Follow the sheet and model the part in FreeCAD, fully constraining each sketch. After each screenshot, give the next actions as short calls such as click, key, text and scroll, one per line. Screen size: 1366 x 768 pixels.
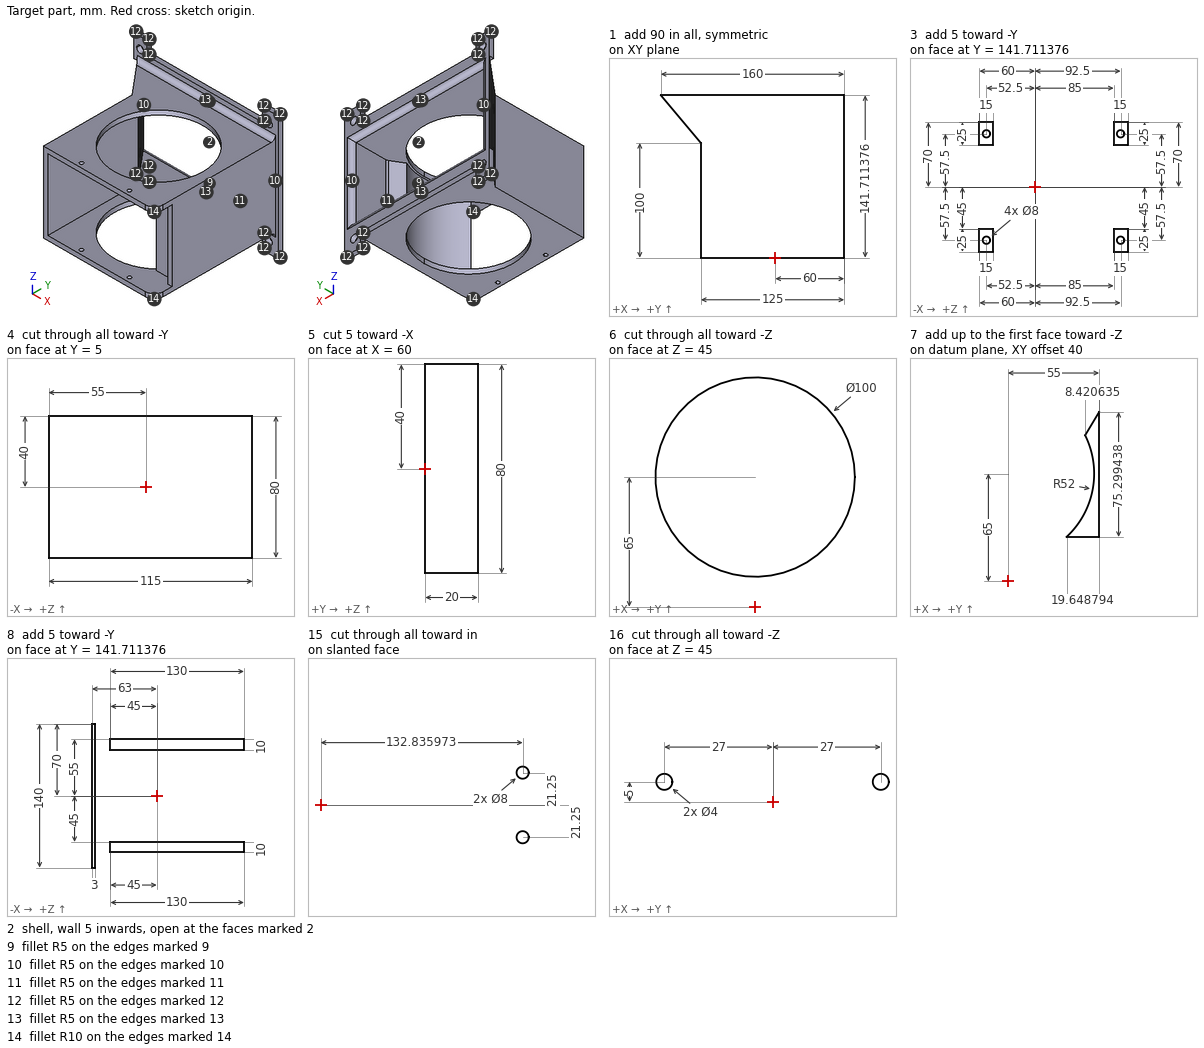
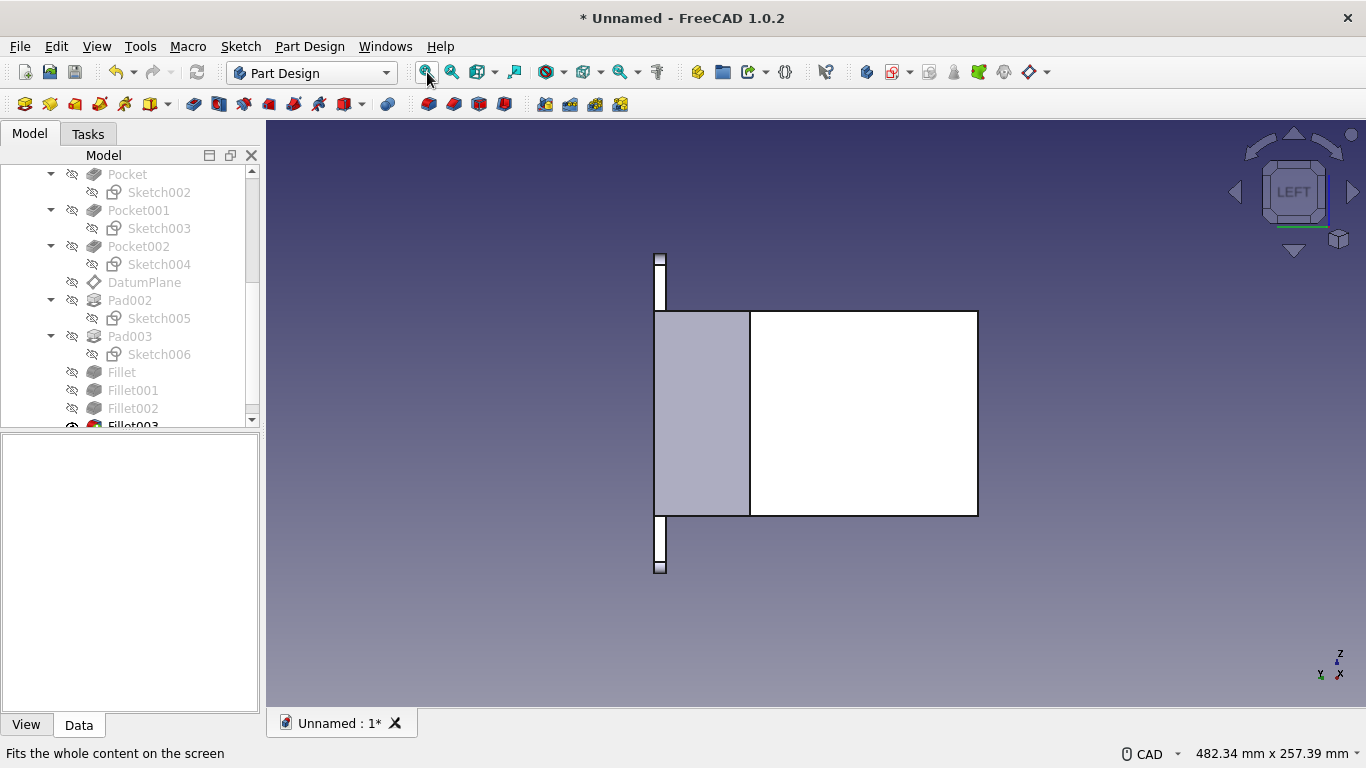
key(v)
key(3)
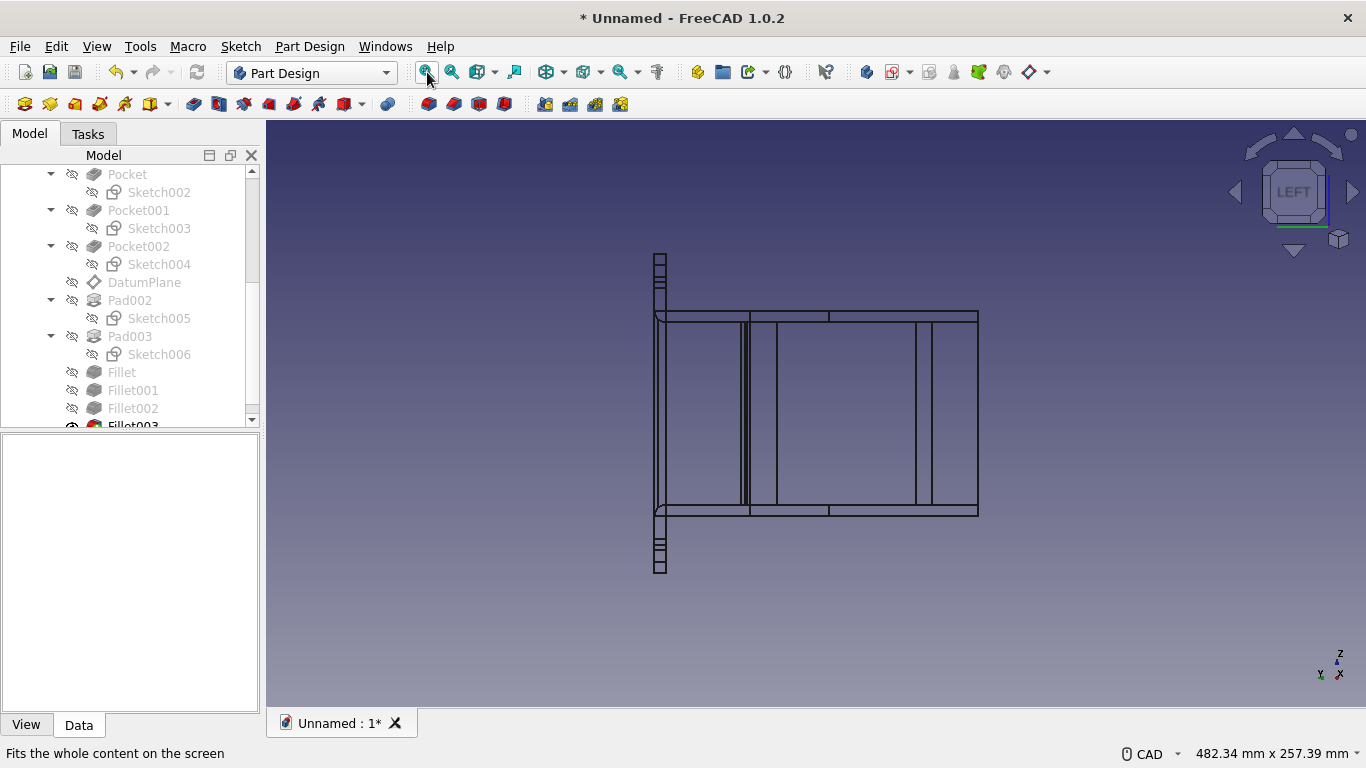
key(0)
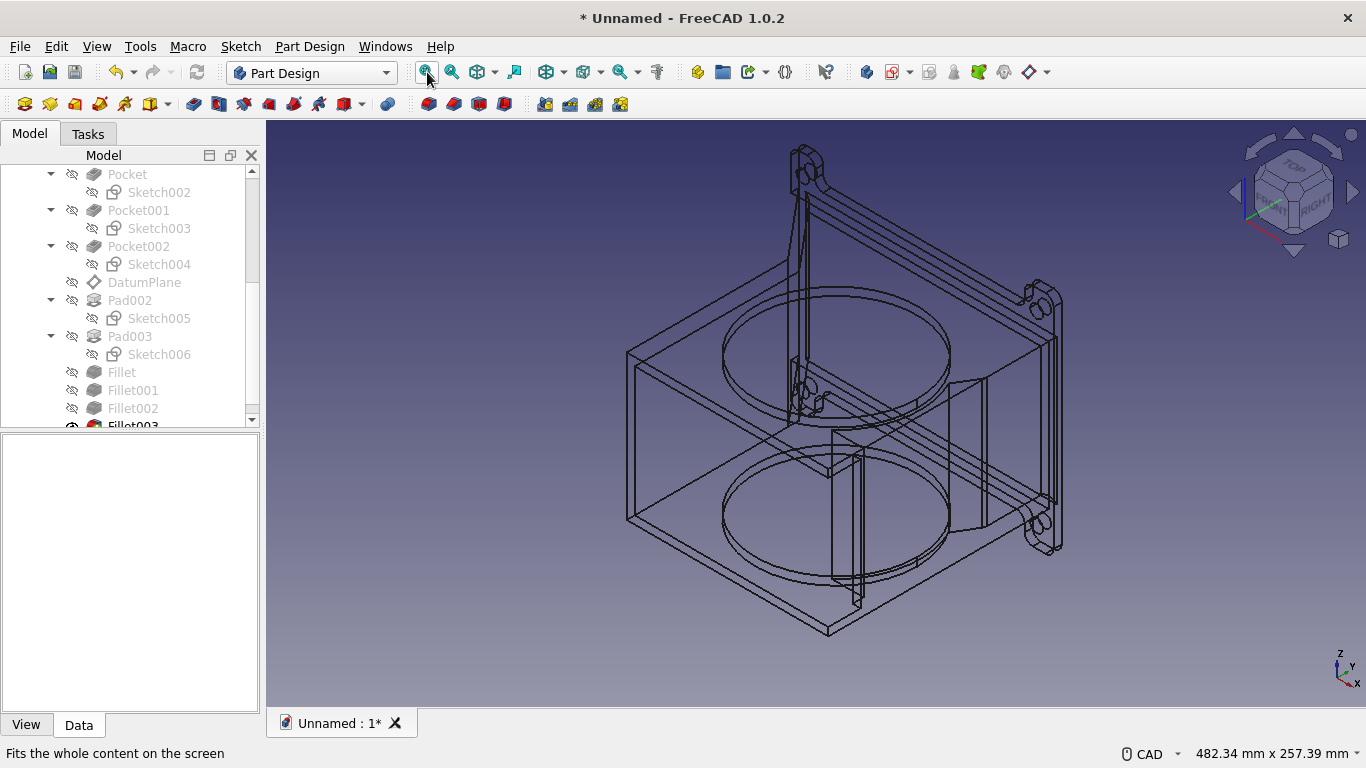
click(923, 436)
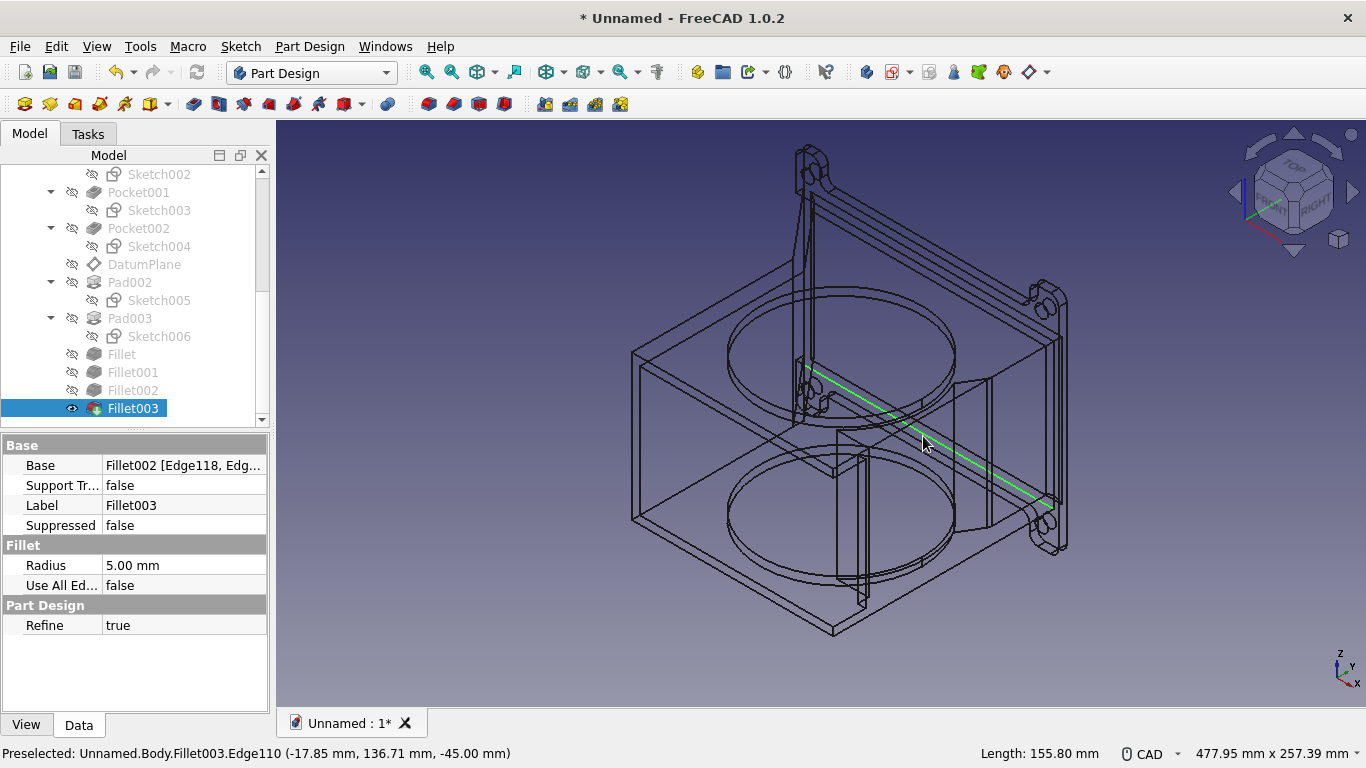
click(928, 268, ctrl)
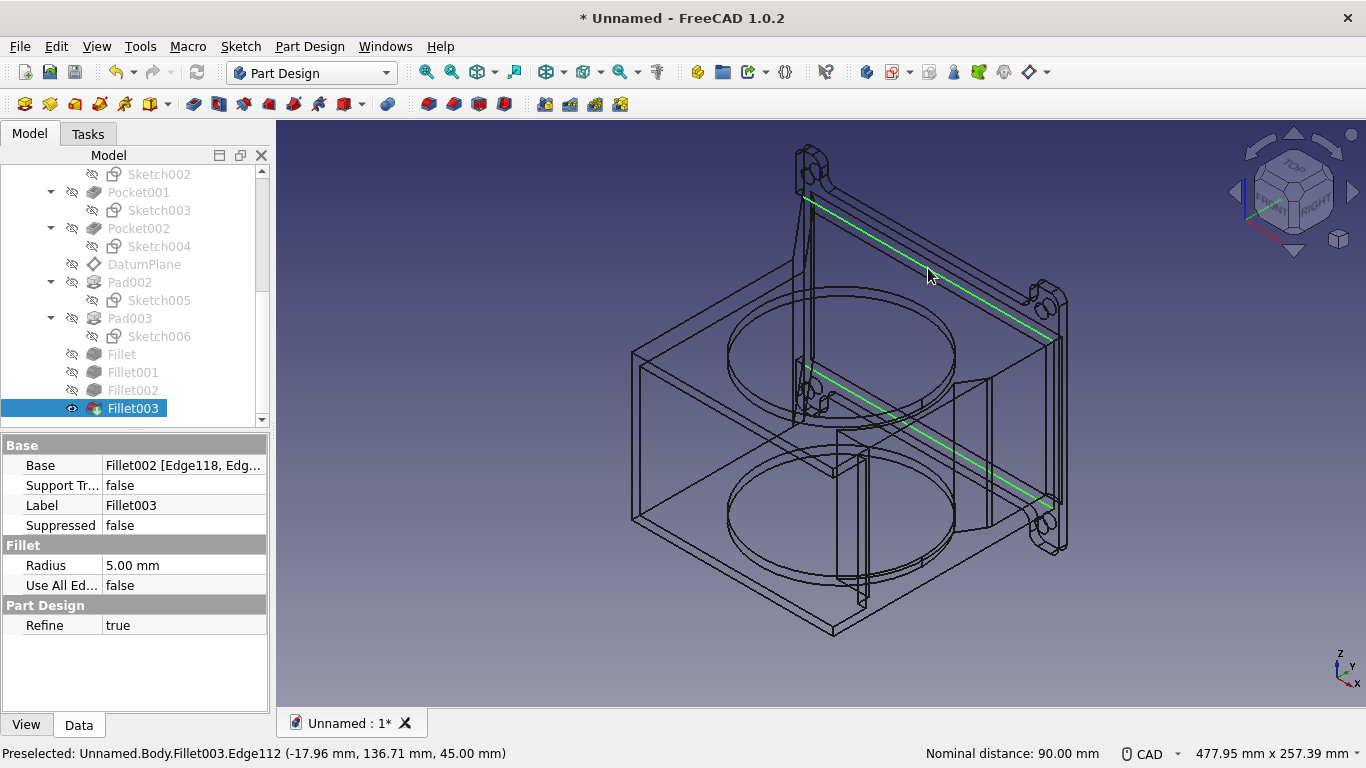
key(v)
key(1)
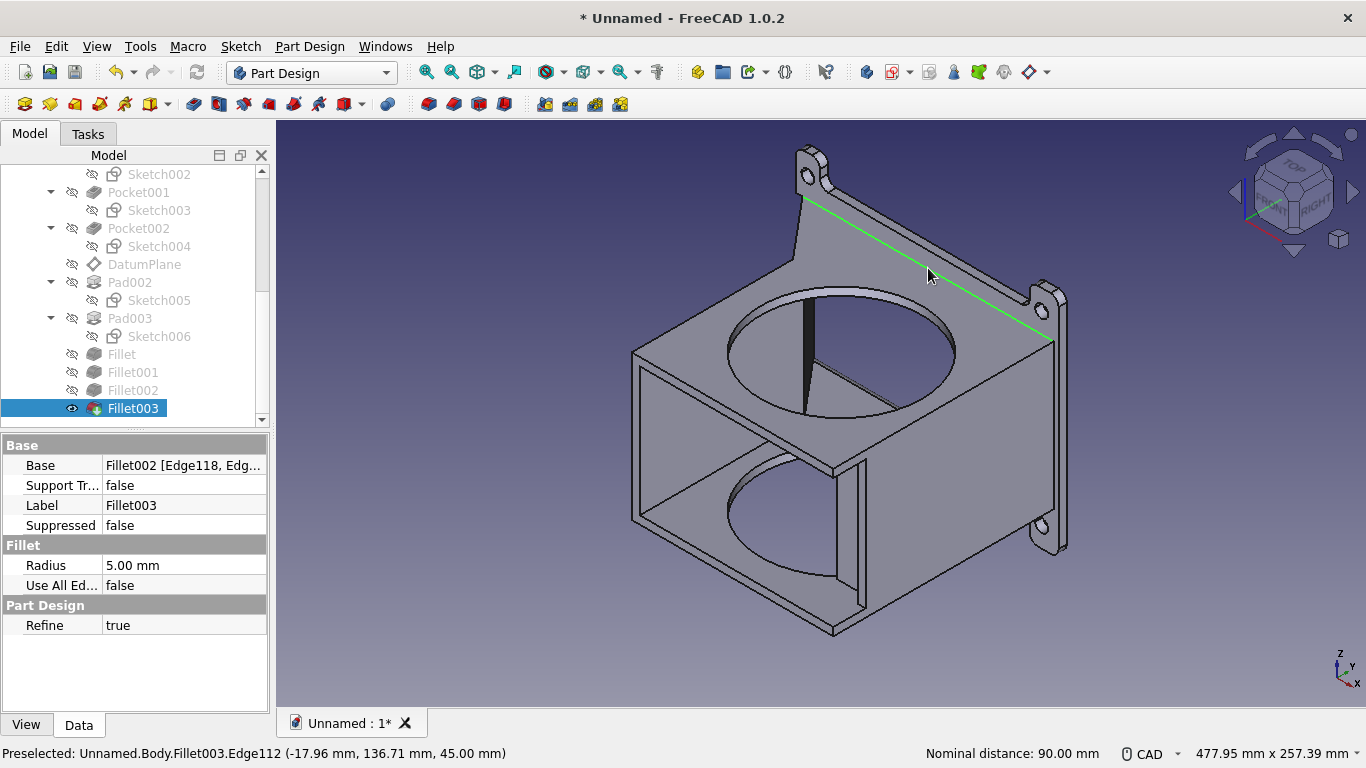
click(429, 104)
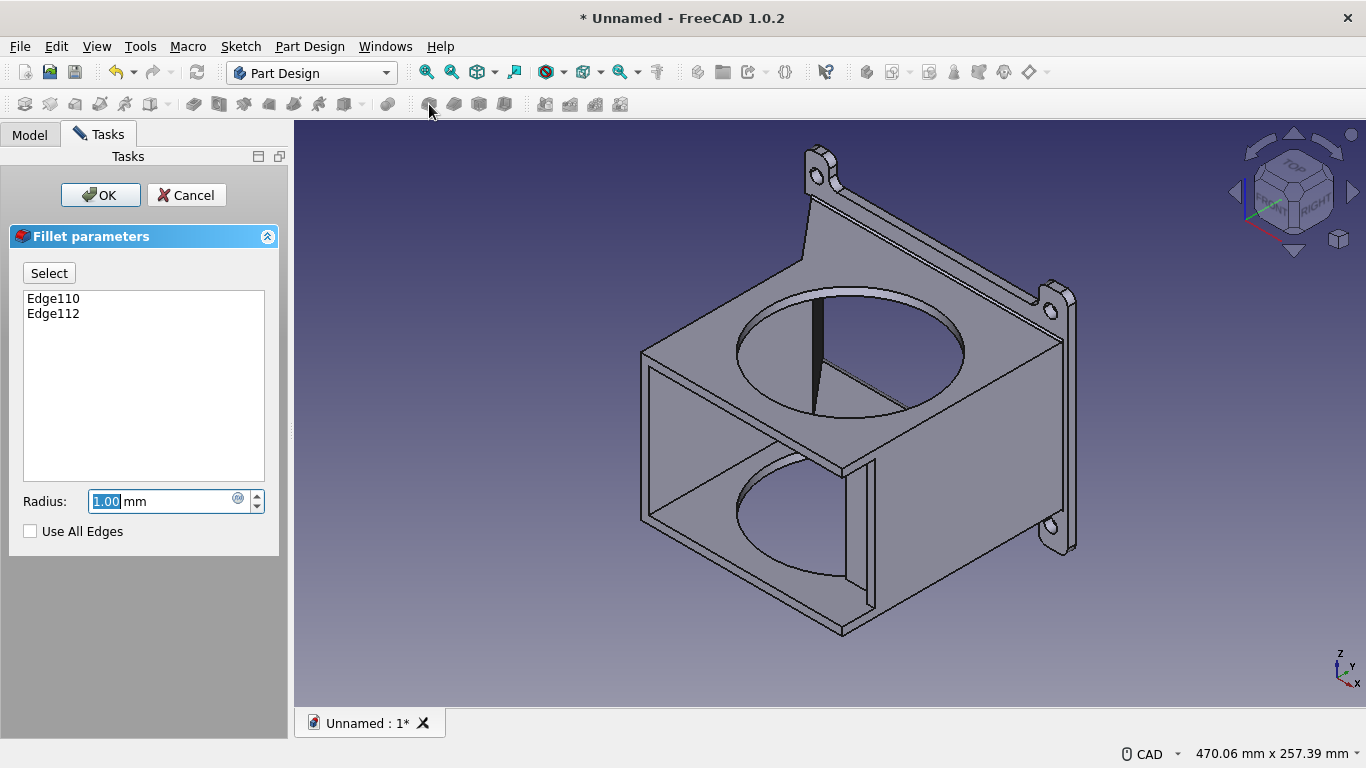
text(5)
key(Tab)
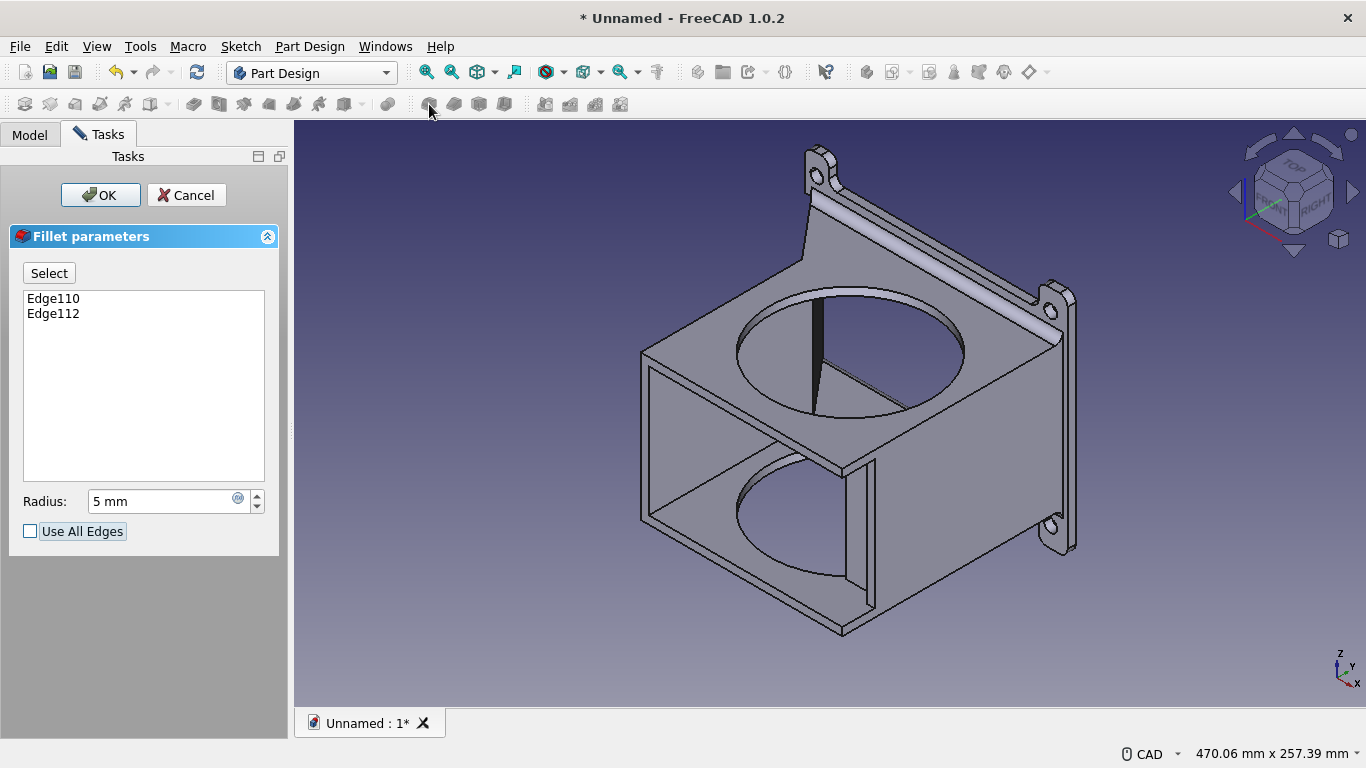
click(101, 195)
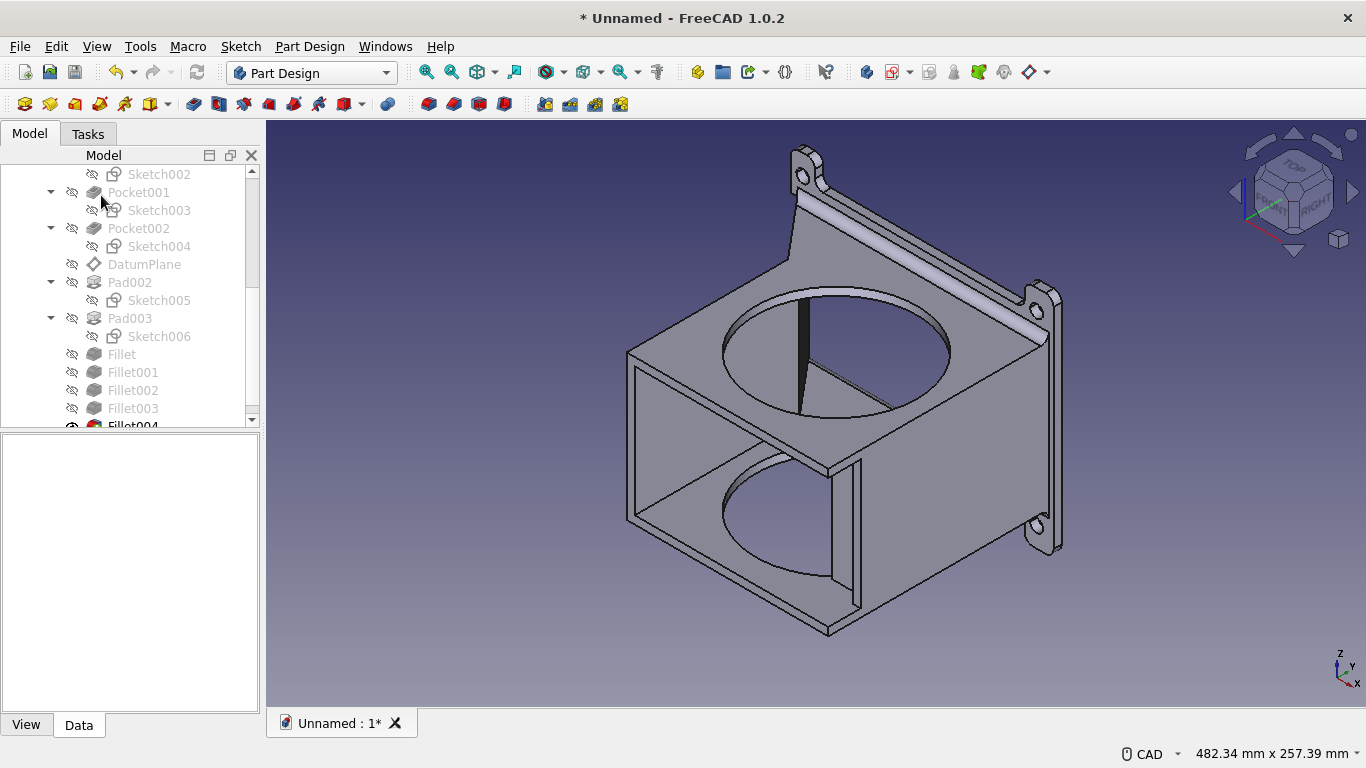
click(828, 474)